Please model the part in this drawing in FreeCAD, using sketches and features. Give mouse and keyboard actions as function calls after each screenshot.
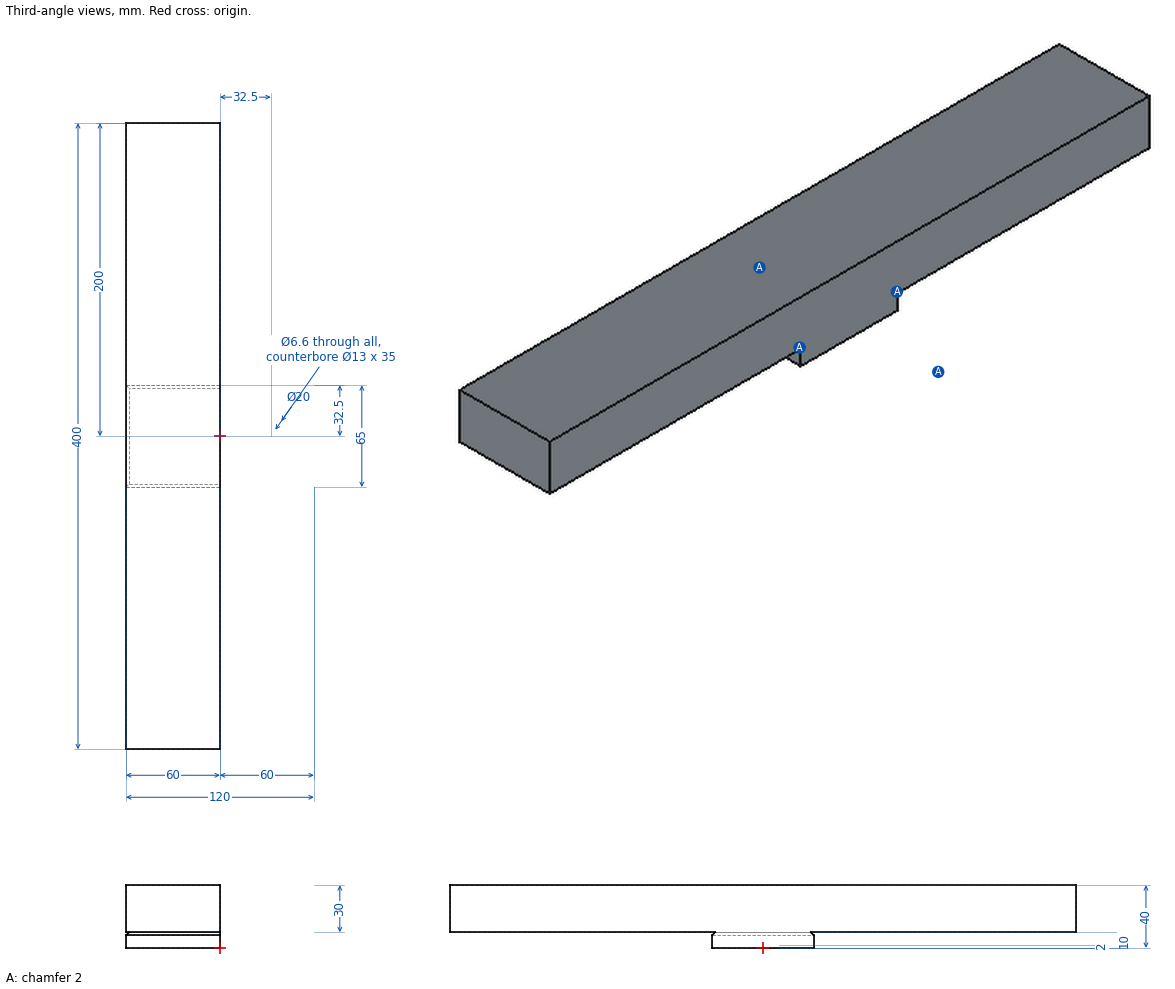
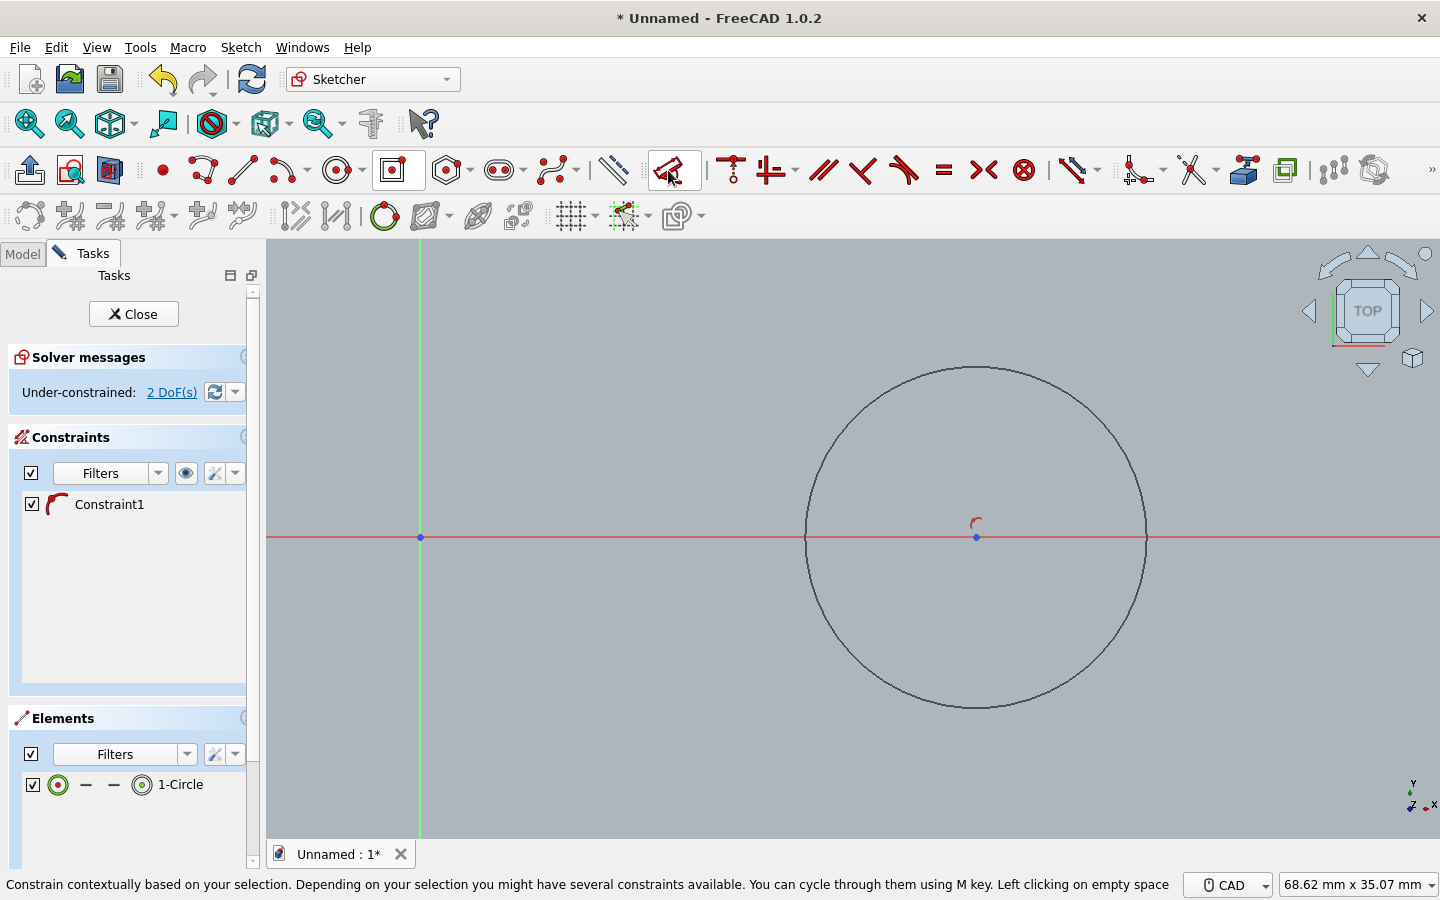
click(1096, 416)
click(1118, 393)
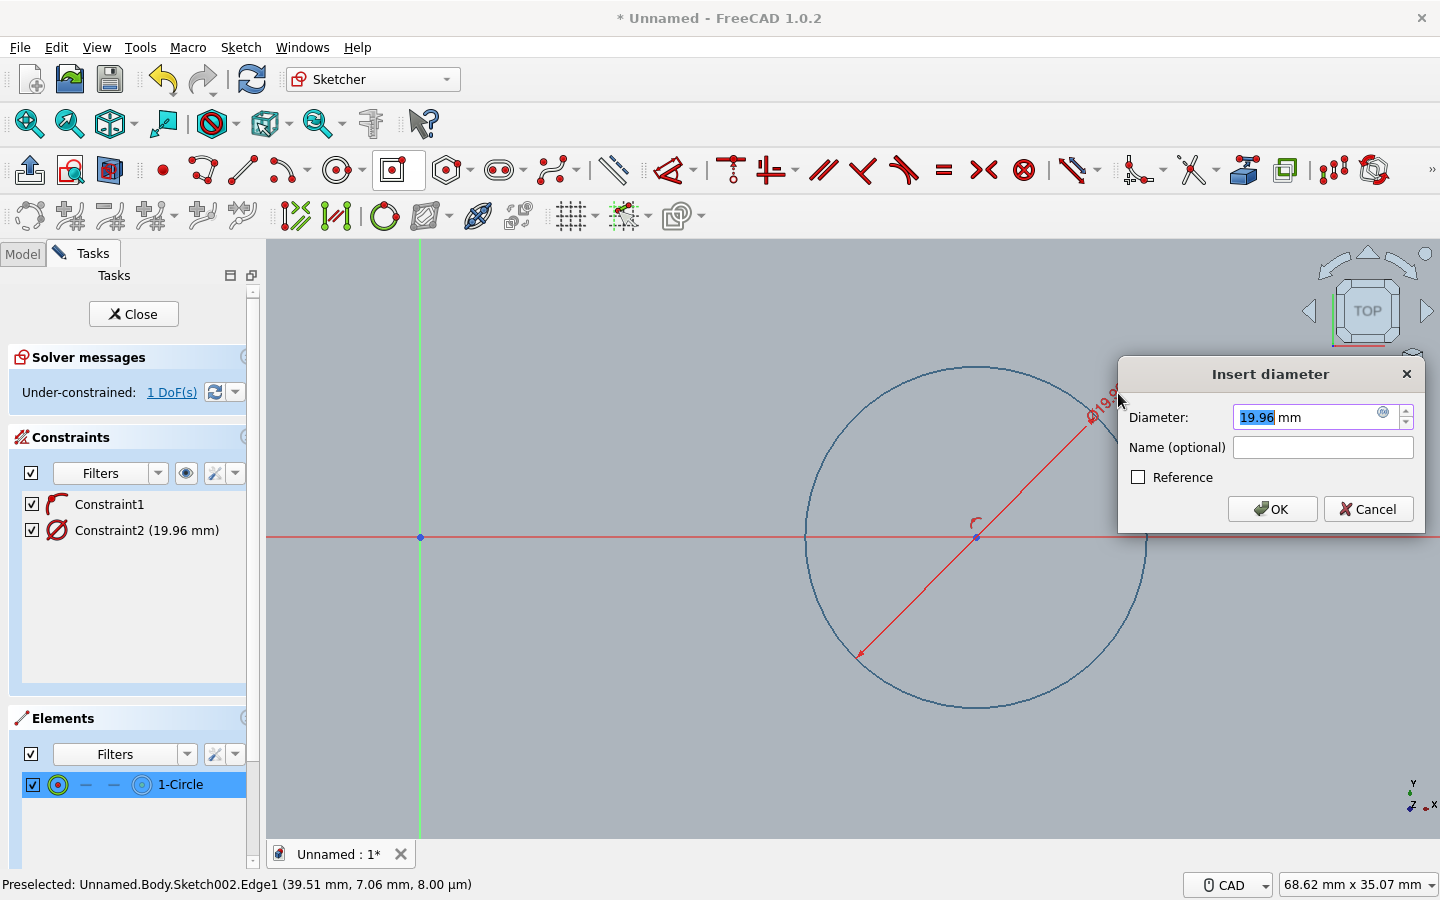
text(20)
key(Return)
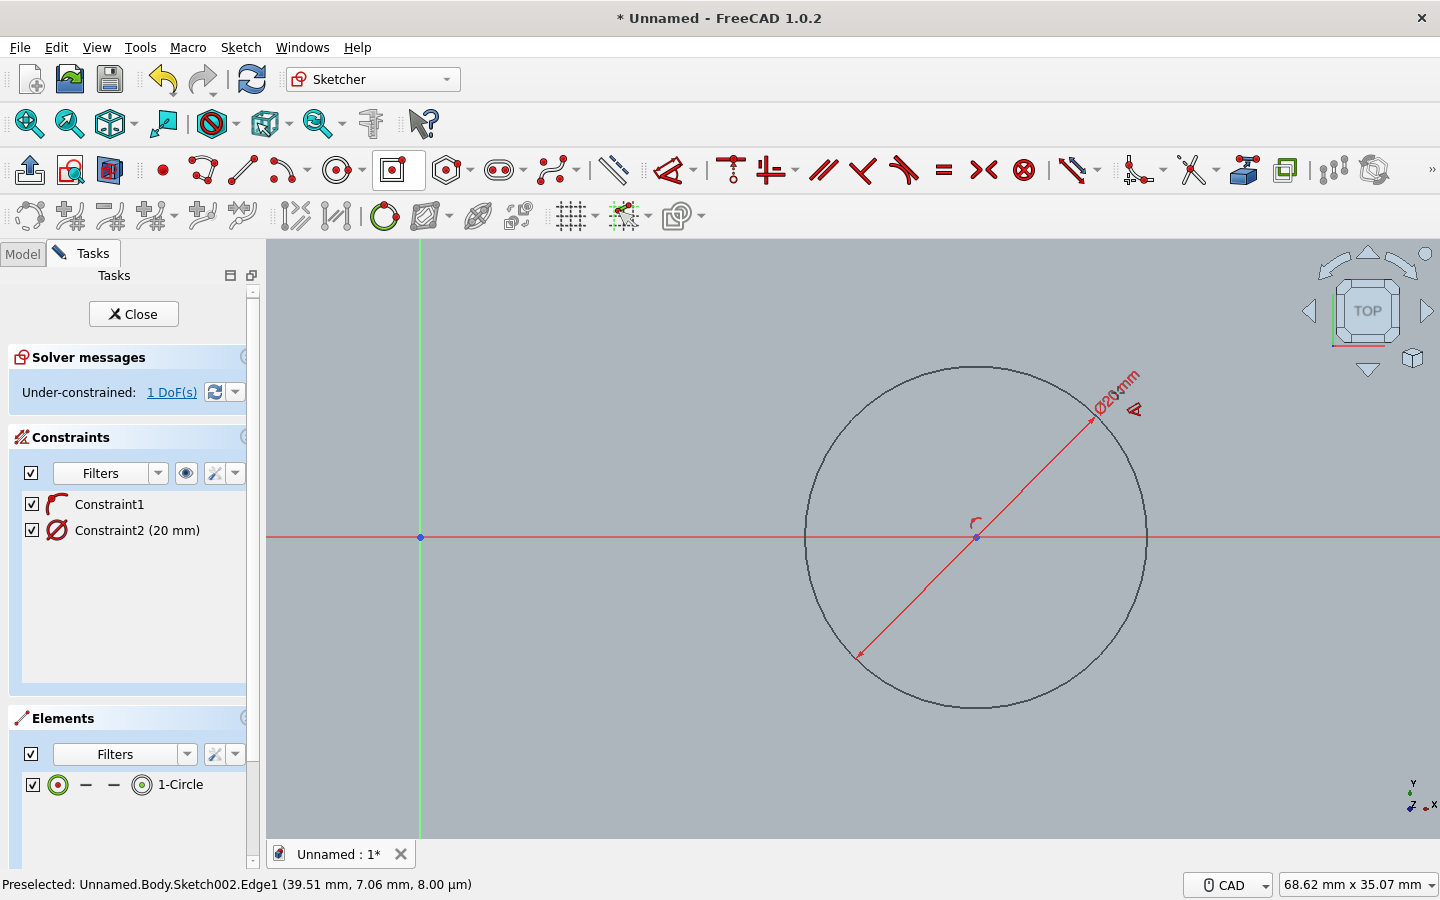
click(976, 537)
click(698, 571)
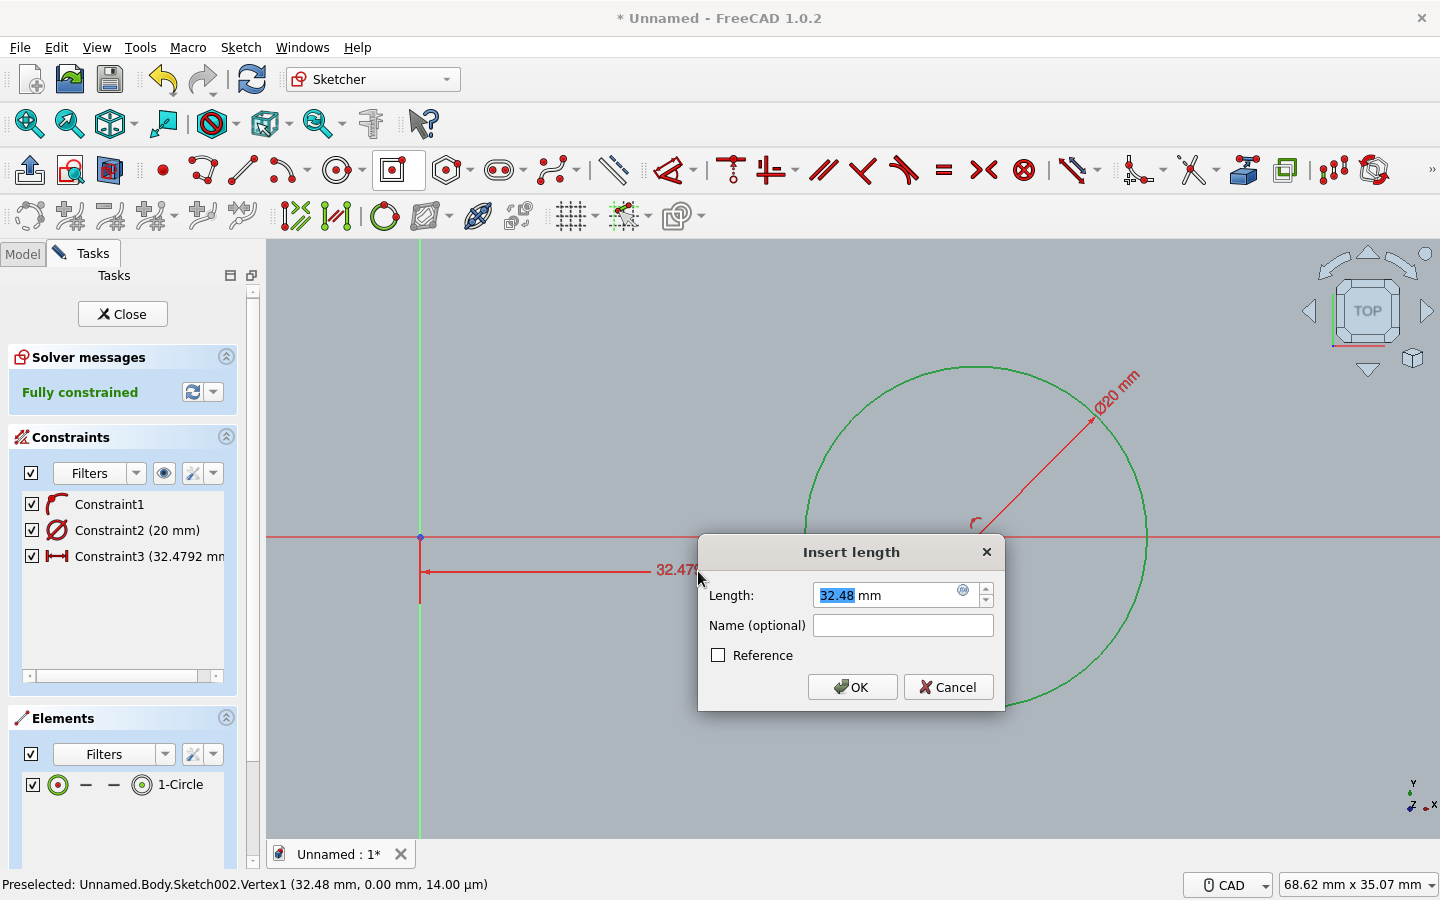
text(32.5)
key(Return)
key(Escape)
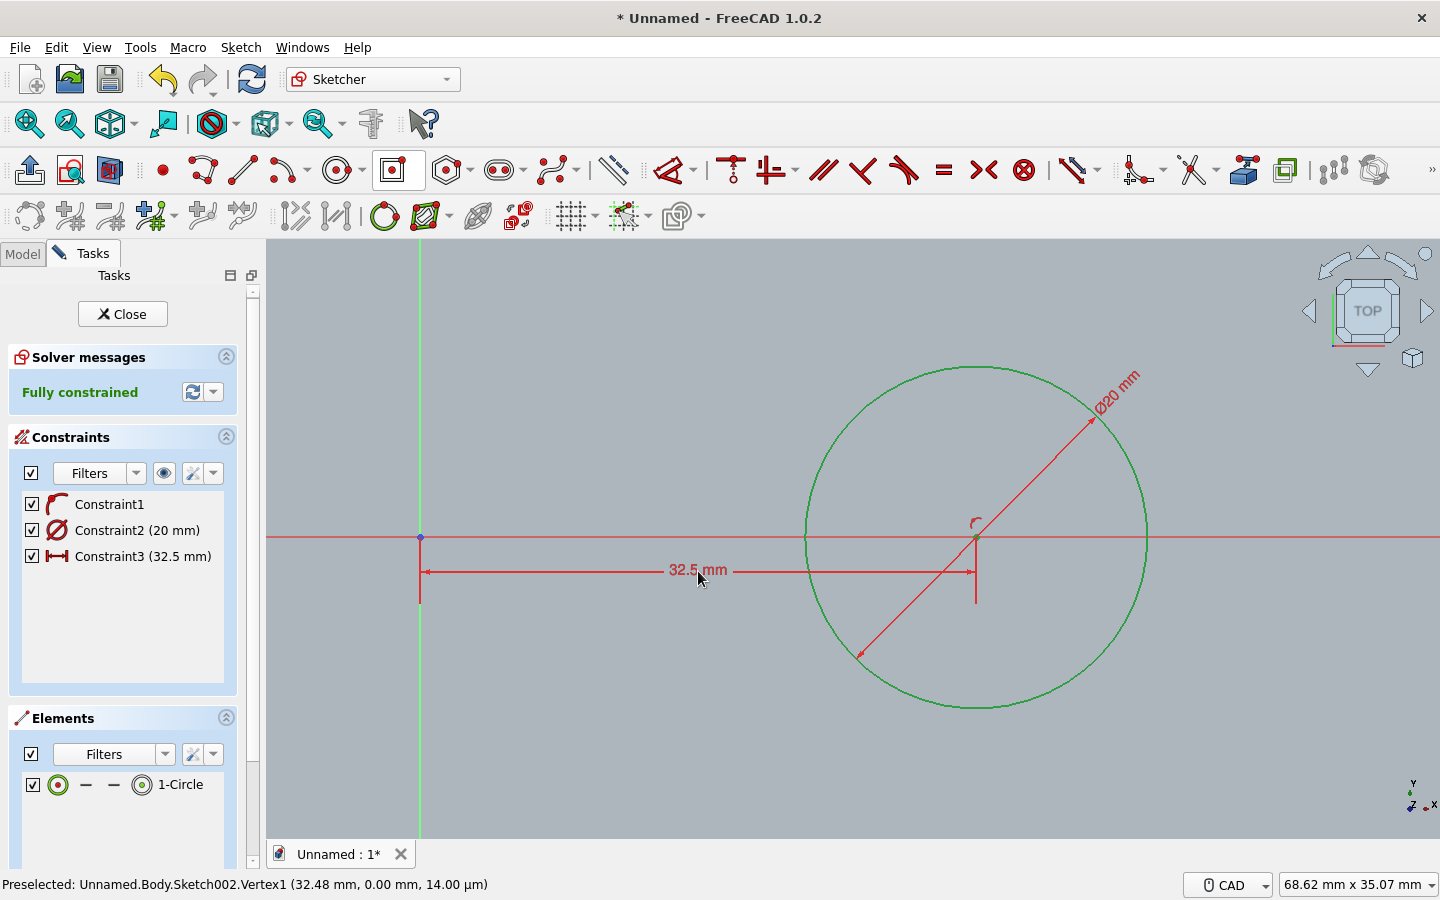
click(123, 314)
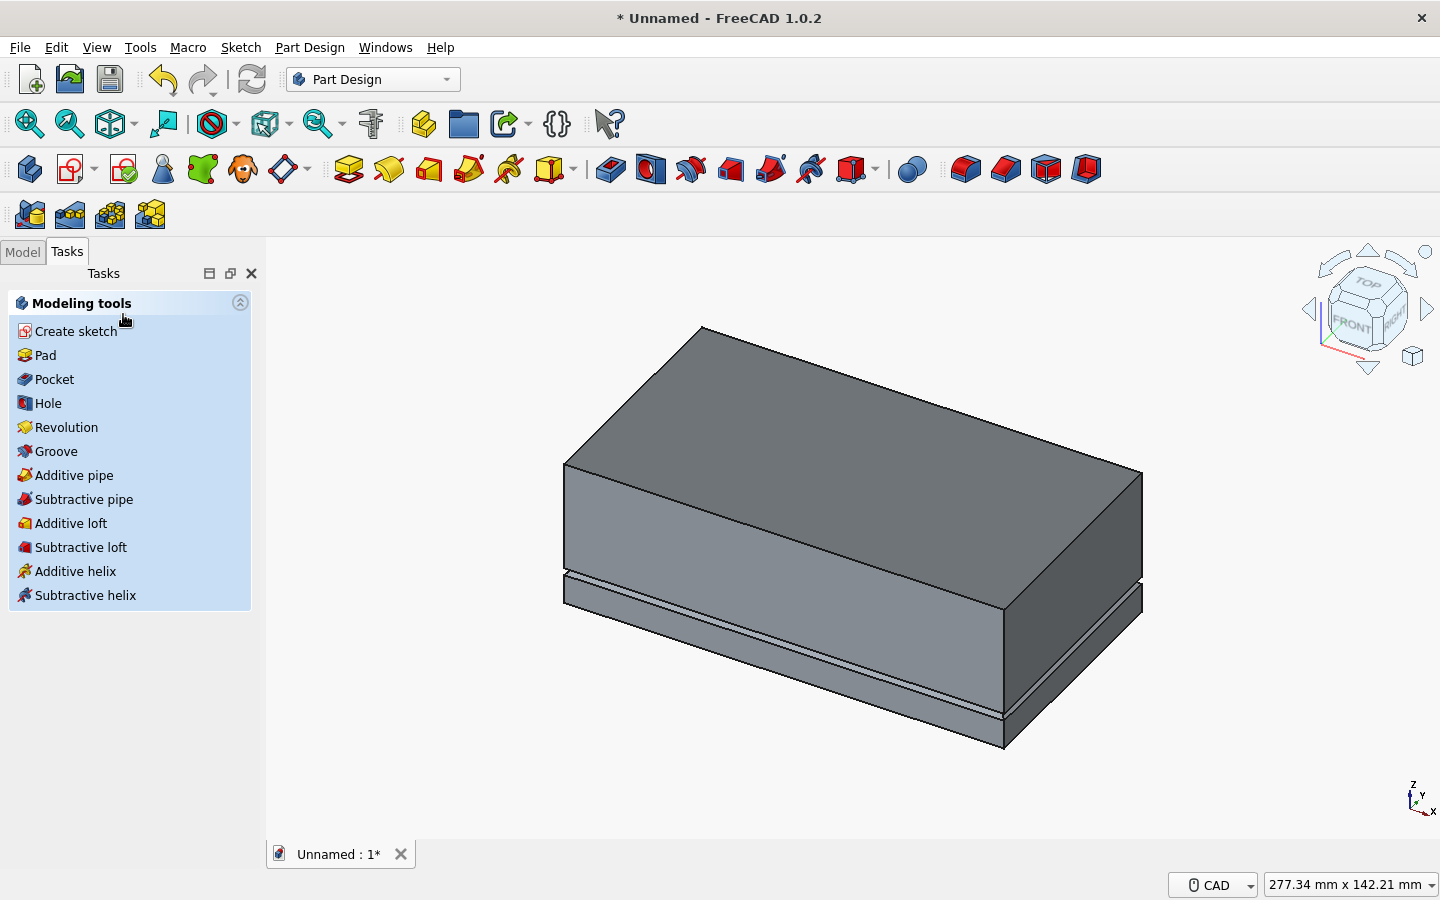
click(612, 170)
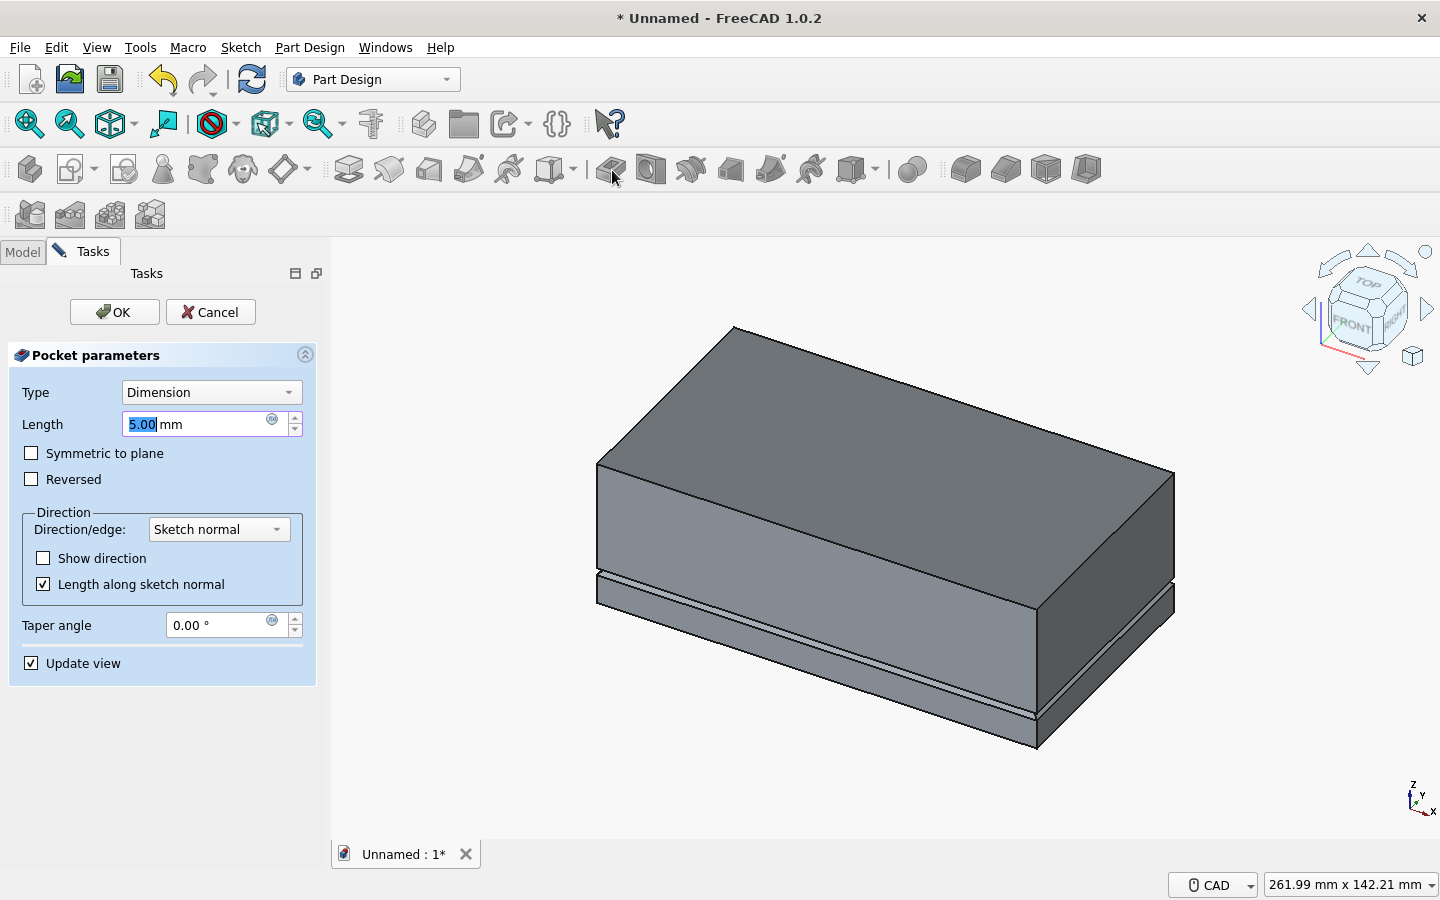
text(2)
key(Tab)